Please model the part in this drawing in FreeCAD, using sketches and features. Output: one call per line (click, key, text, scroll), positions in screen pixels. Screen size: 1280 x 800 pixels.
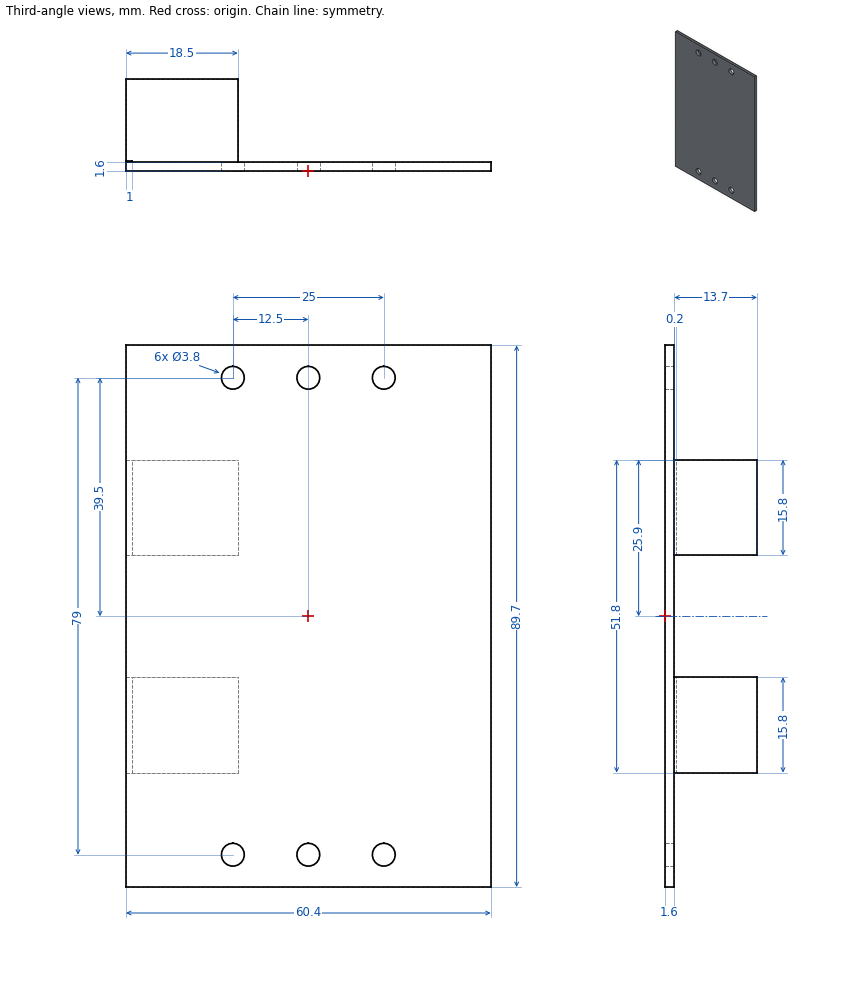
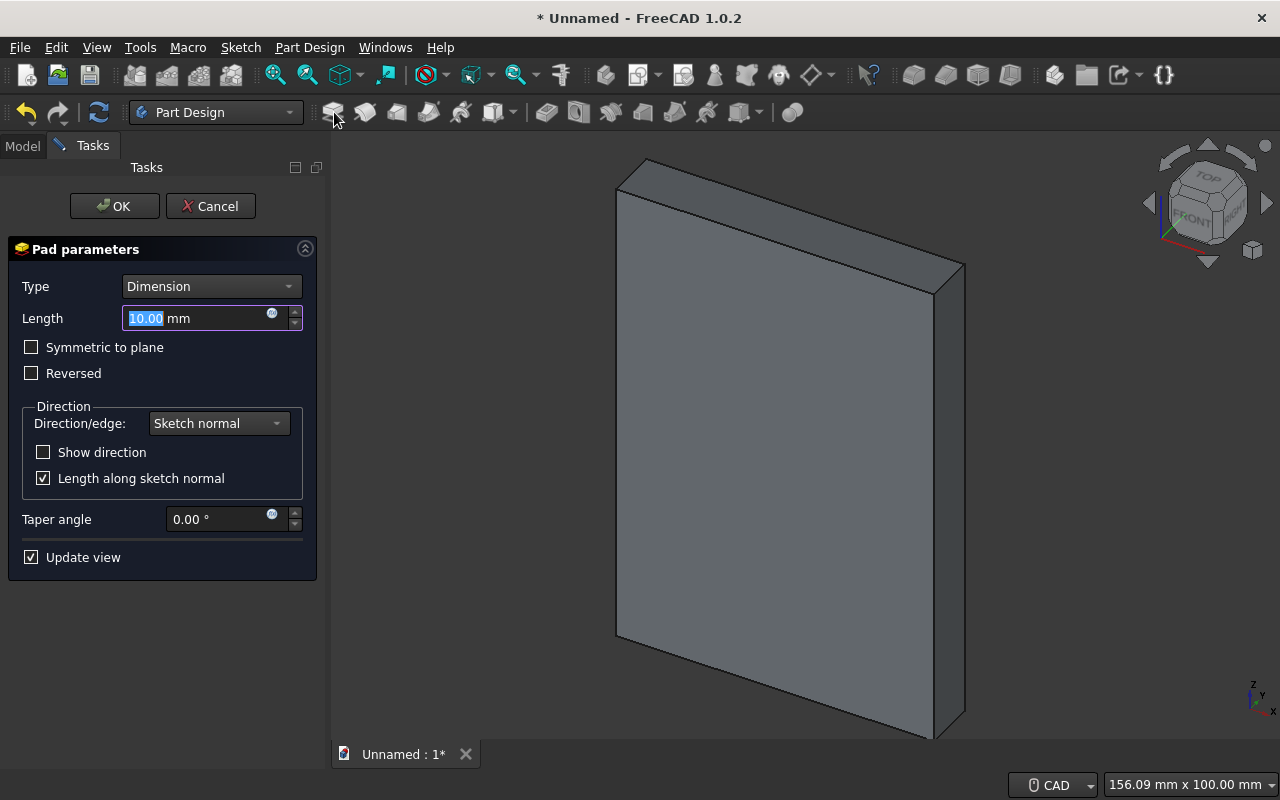
text(1.6)
key(Tab)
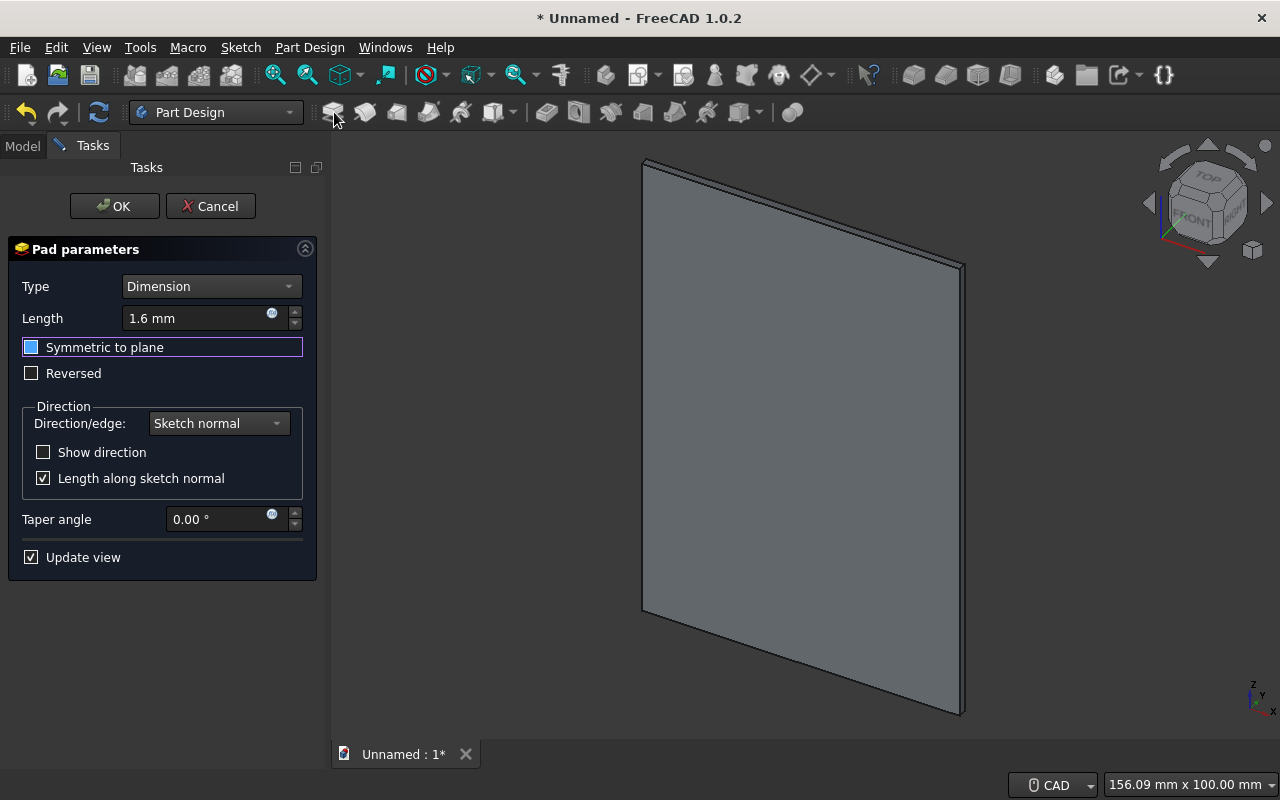
click(30, 373)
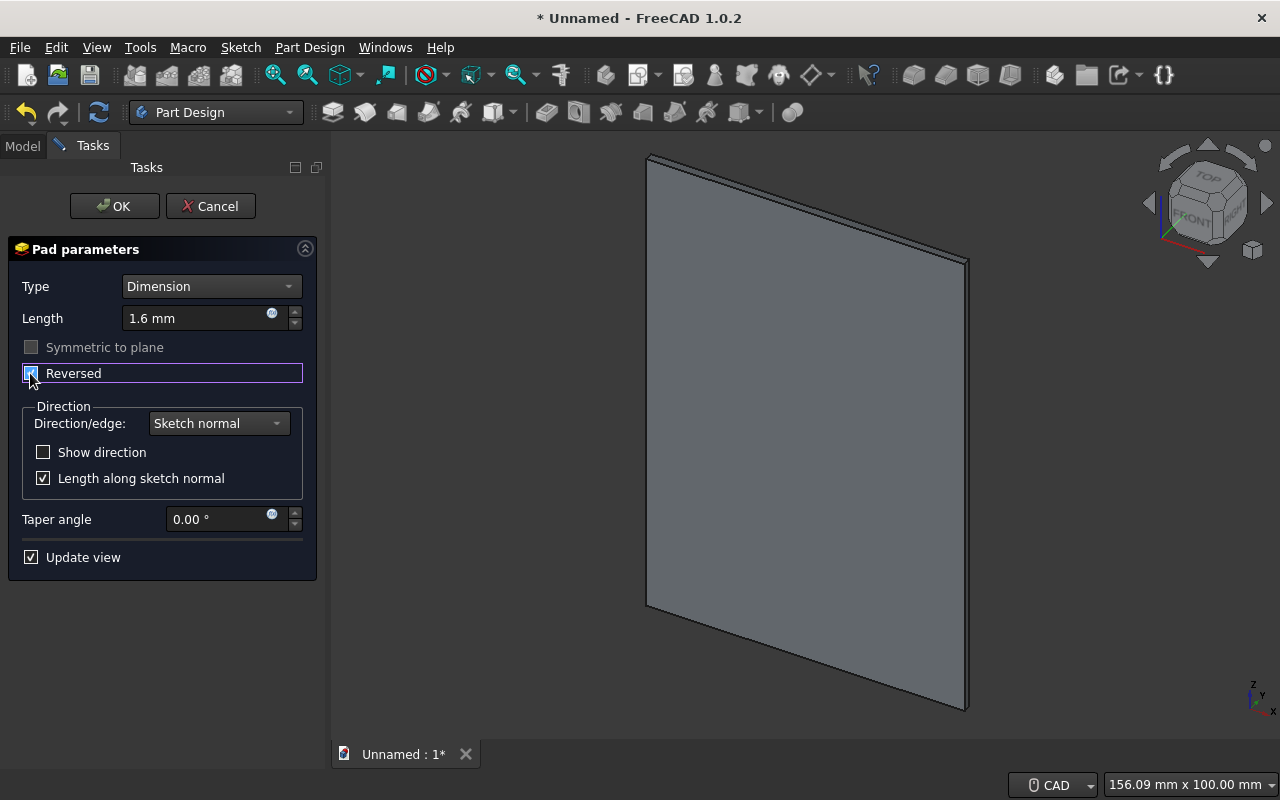
click(115, 206)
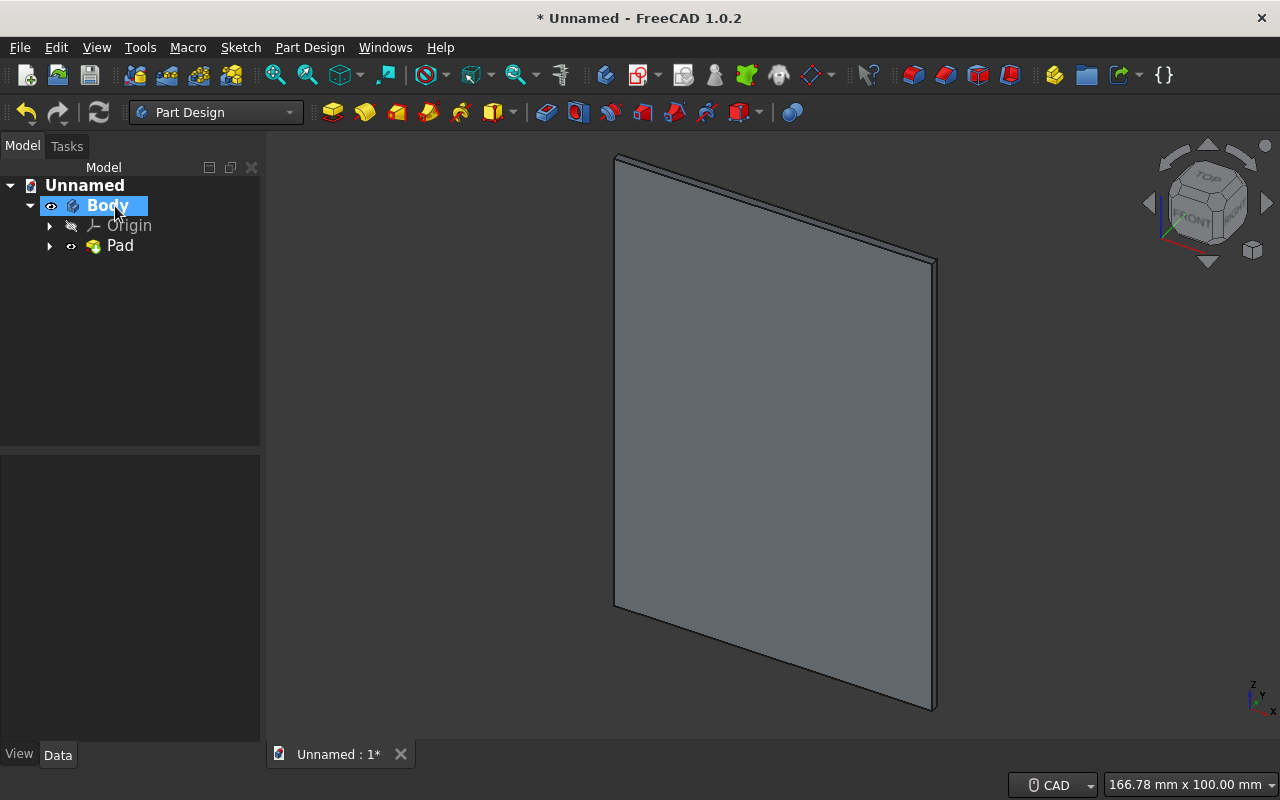
key(4)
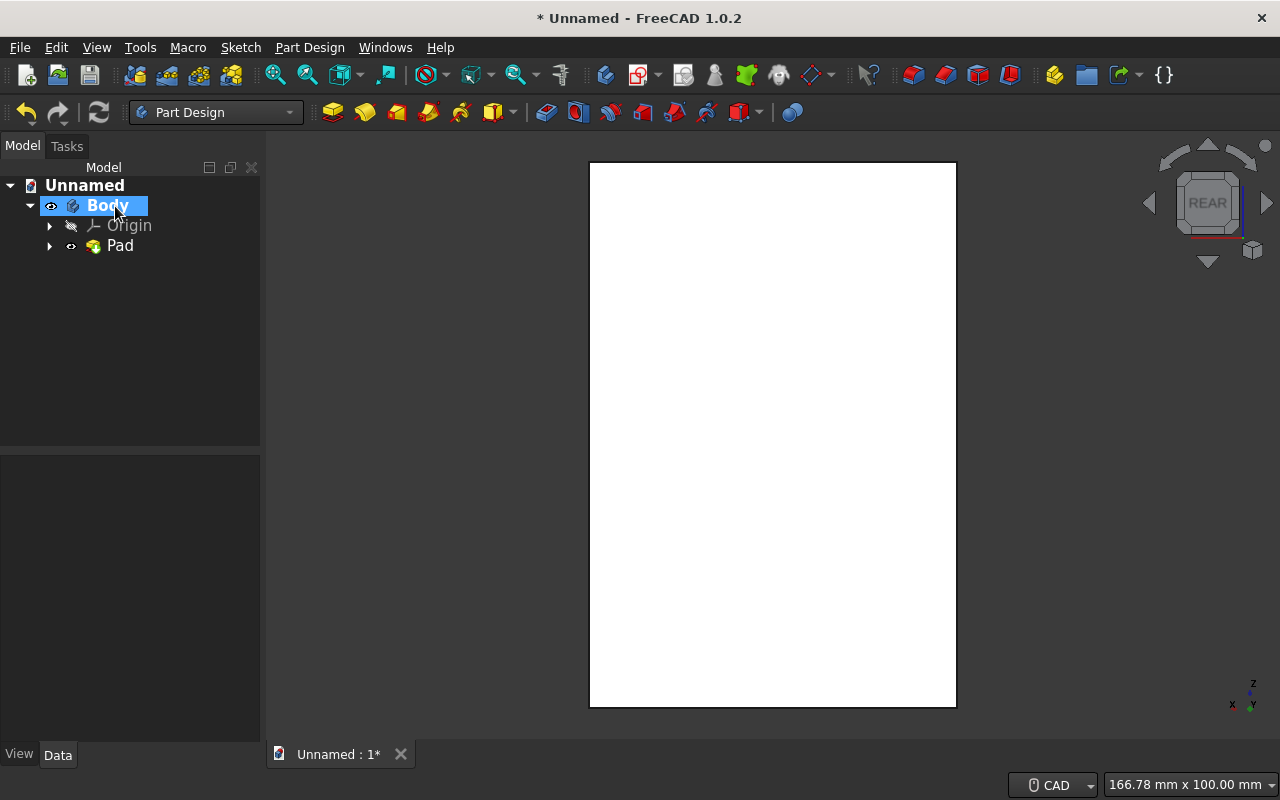
click(773, 356)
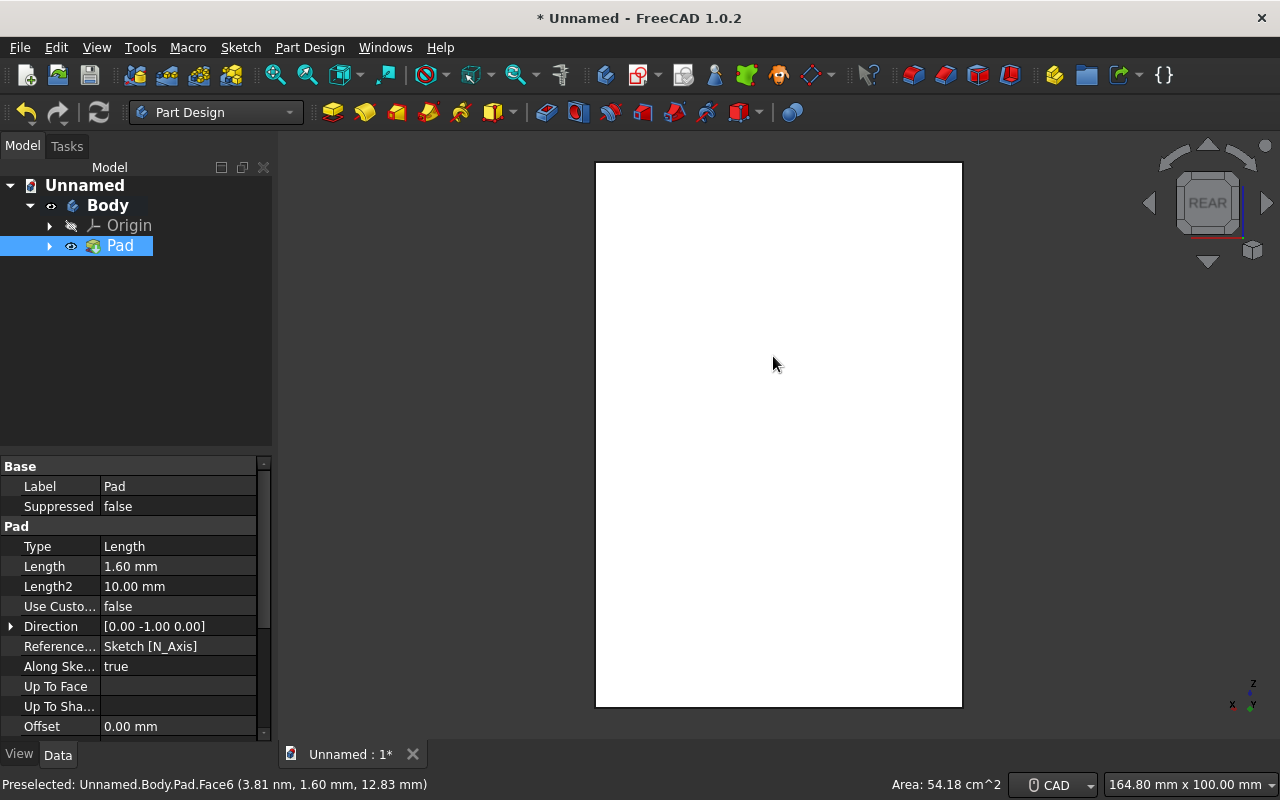
click(638, 76)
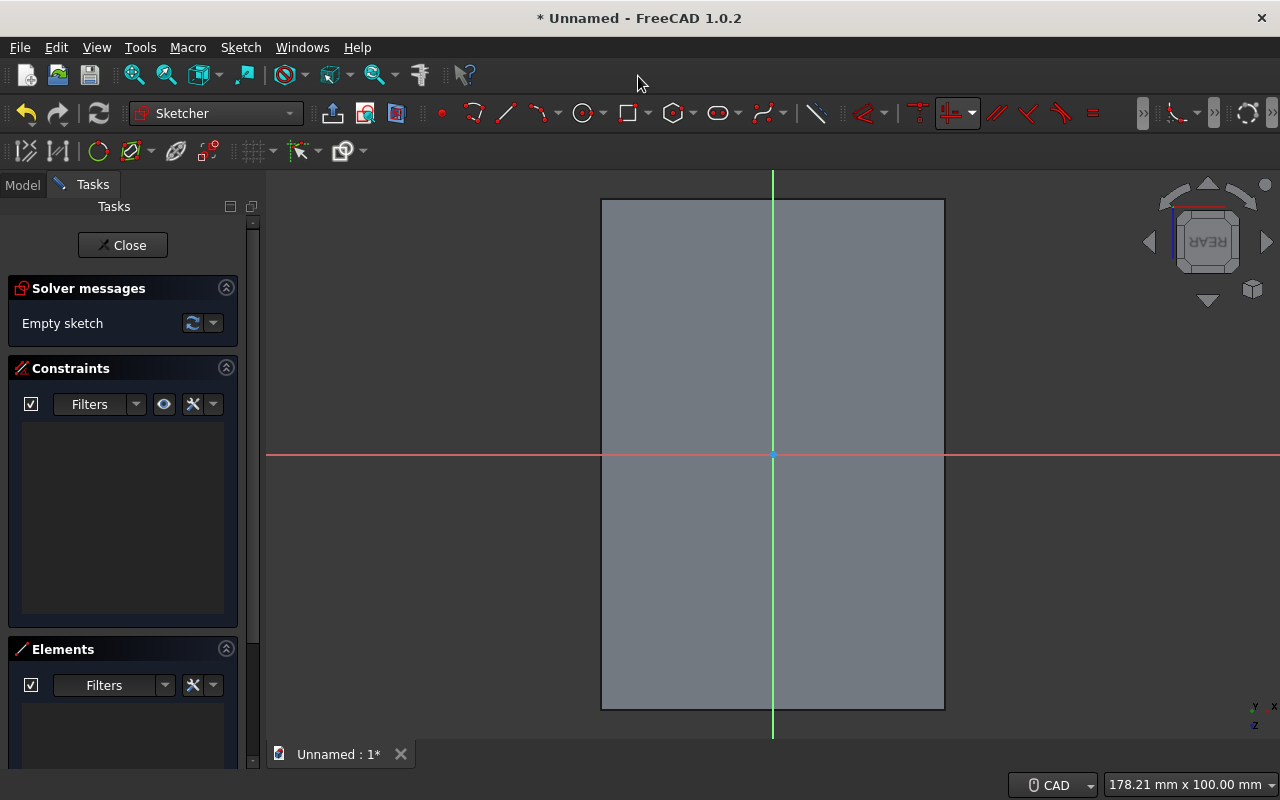
scroll(395, 454, down, 1)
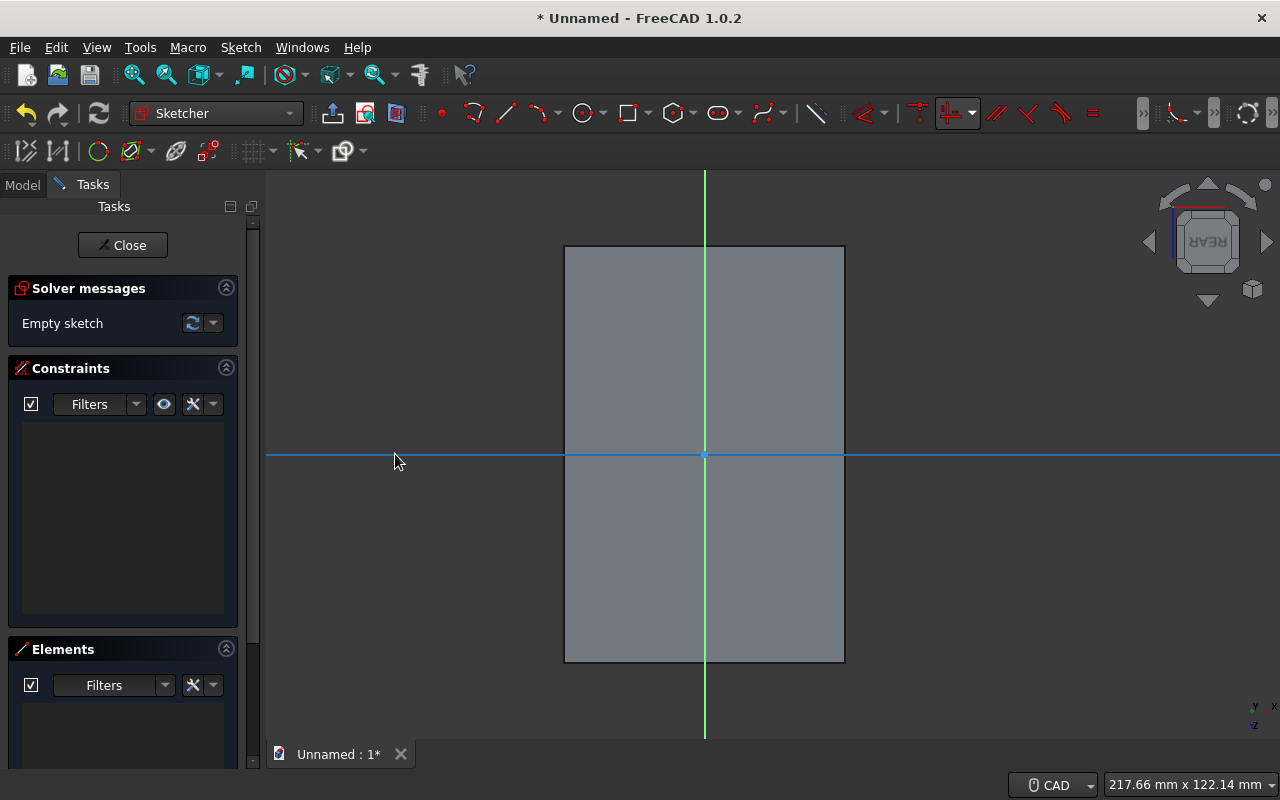
click(584, 114)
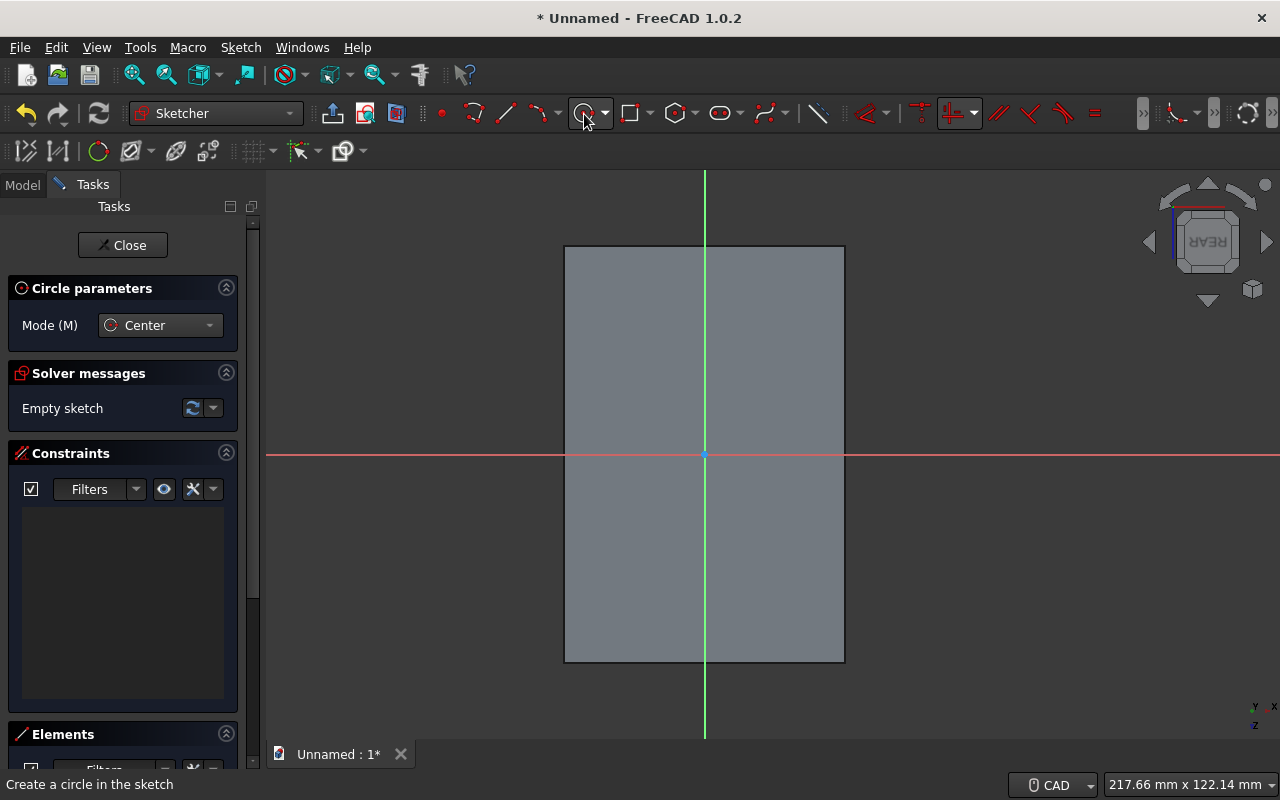
scroll(646, 639, up, 5)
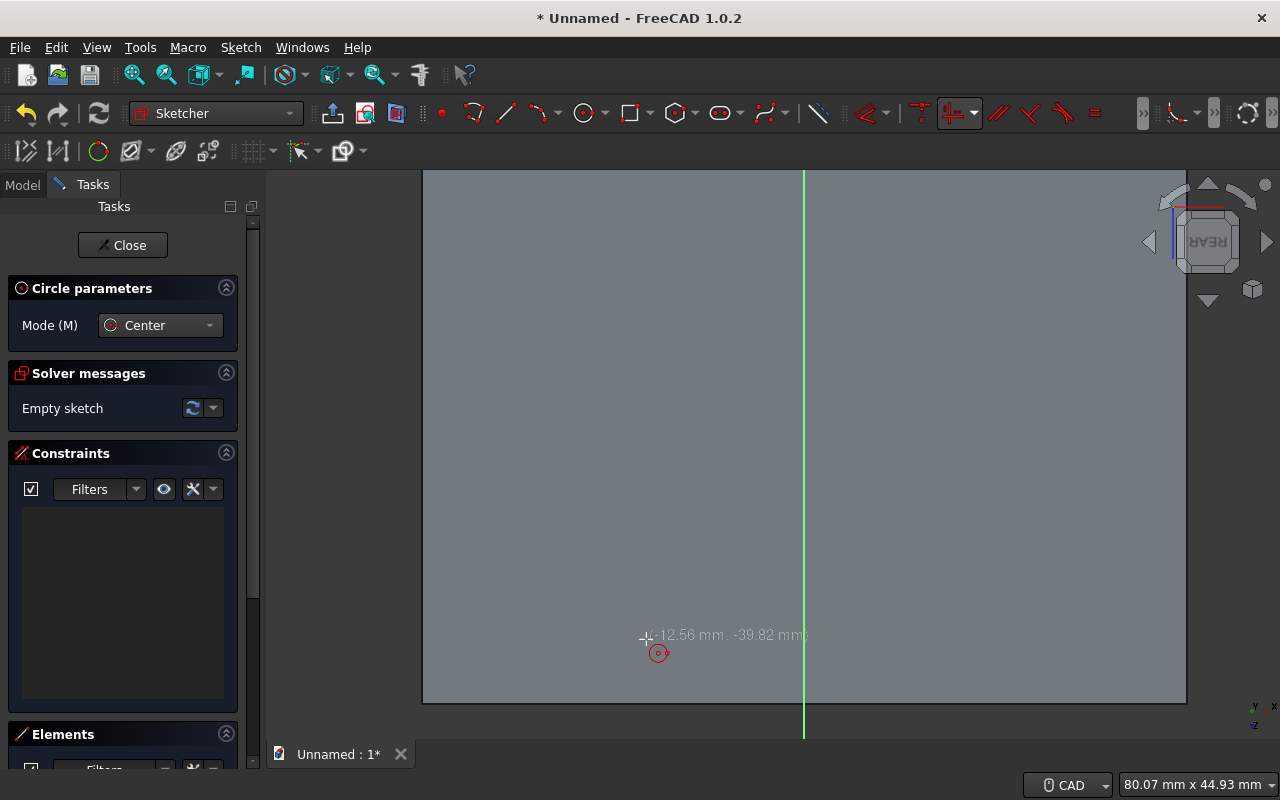
click(646, 636)
move(663, 619)